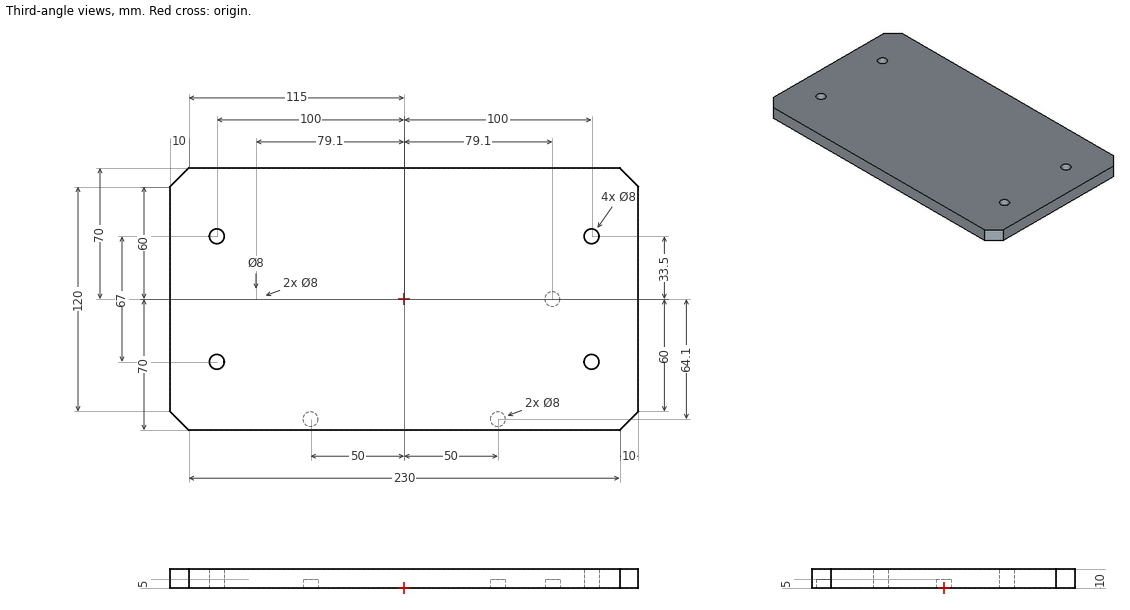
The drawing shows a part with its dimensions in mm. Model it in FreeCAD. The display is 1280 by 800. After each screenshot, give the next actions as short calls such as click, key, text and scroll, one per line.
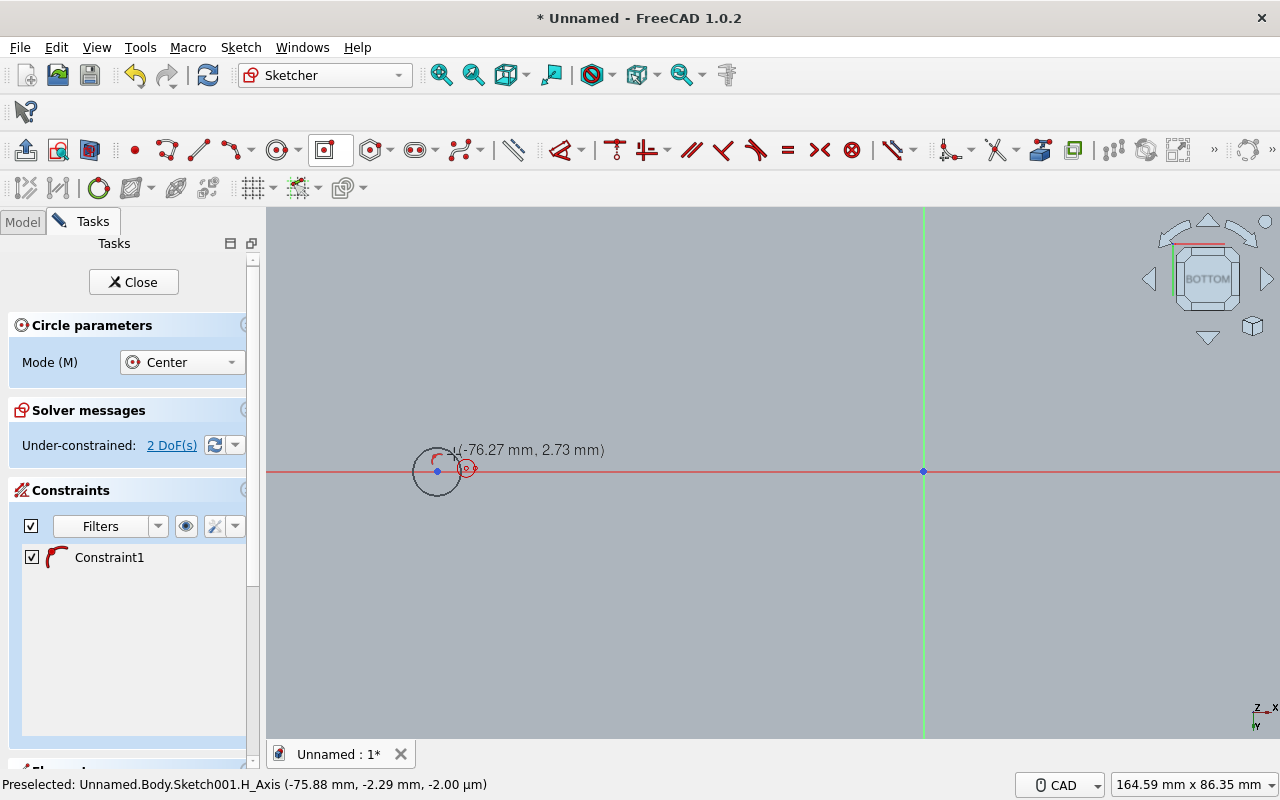
scroll(438, 474, down, 3)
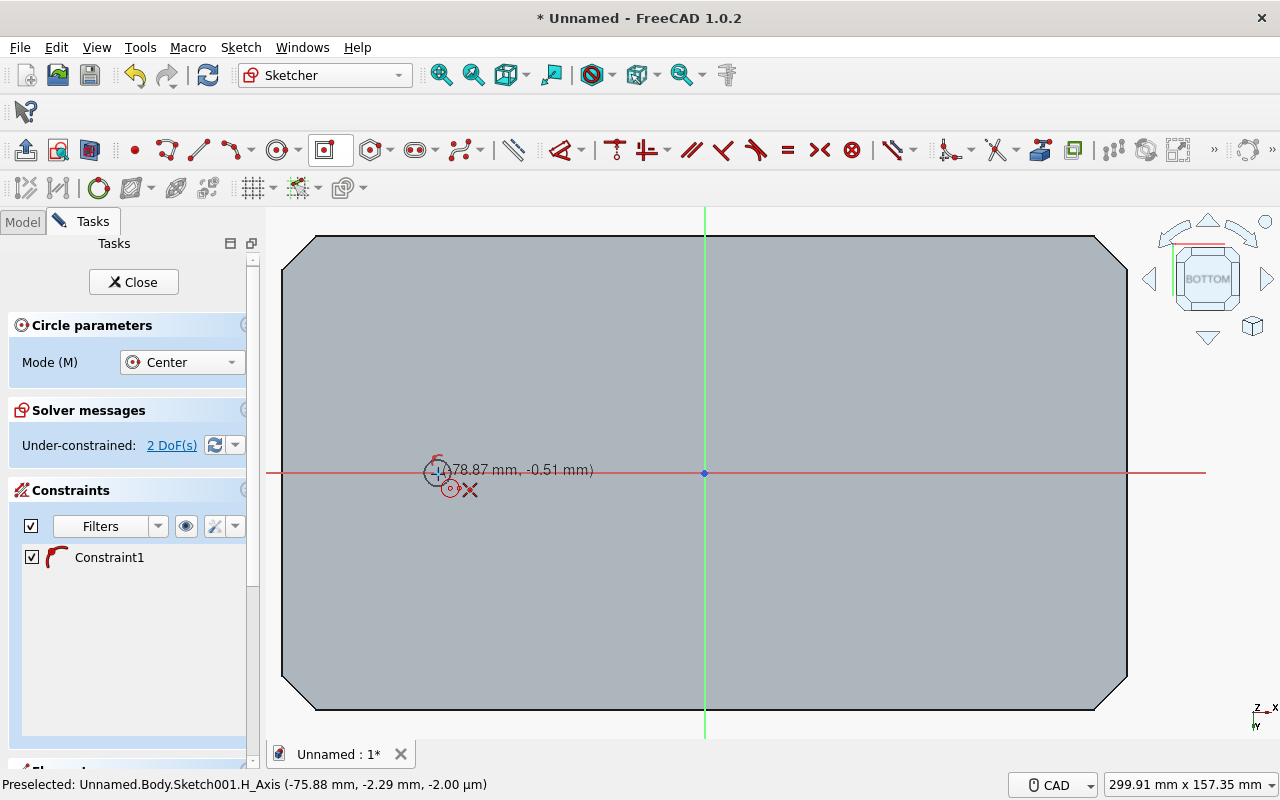
scroll(972, 473, up, 3)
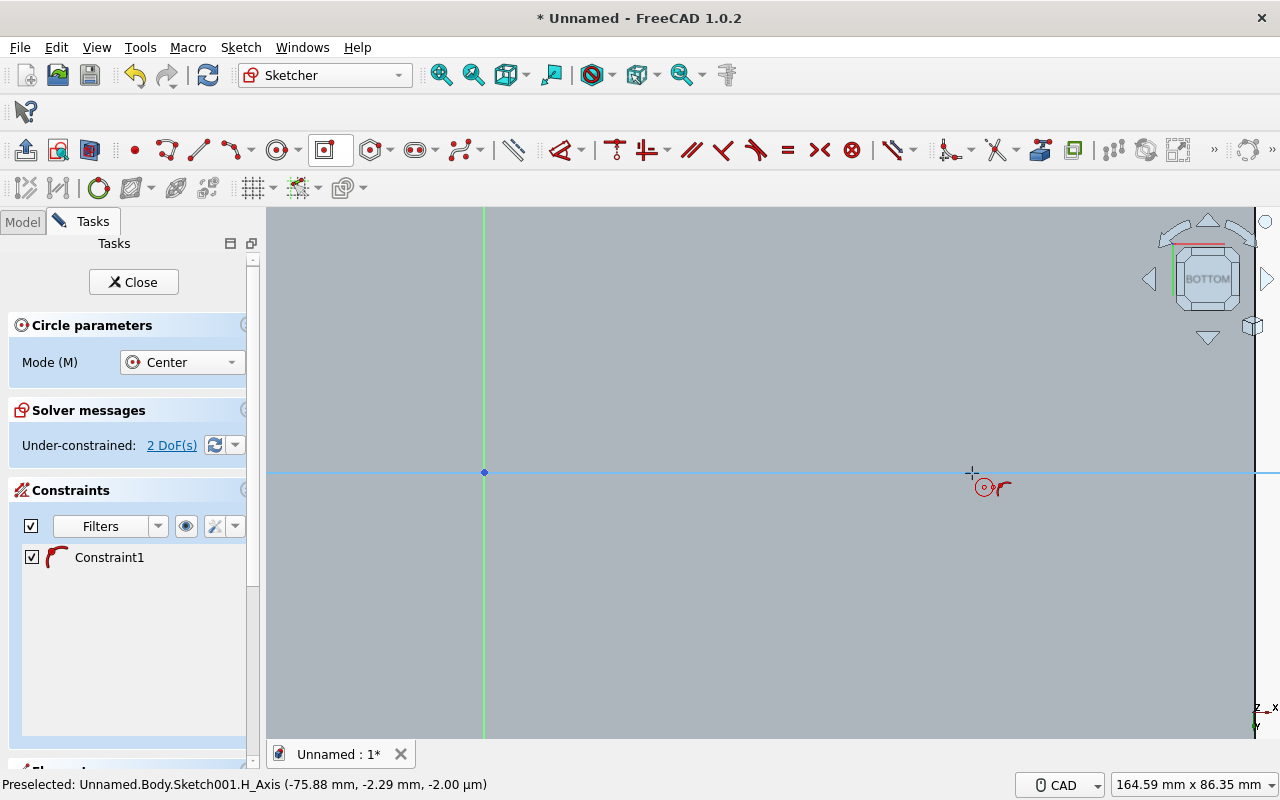
click(972, 473)
click(989, 455)
key(Escape)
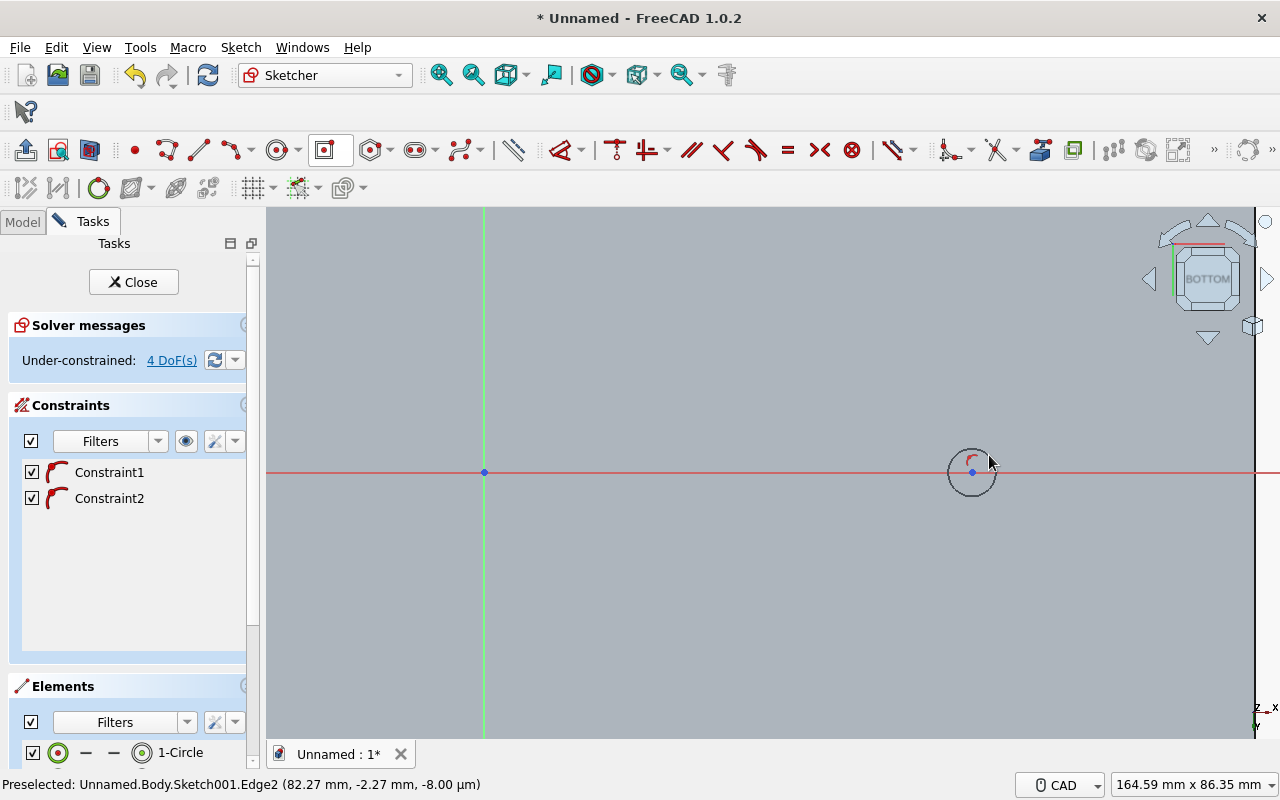
scroll(972, 473, down, 3)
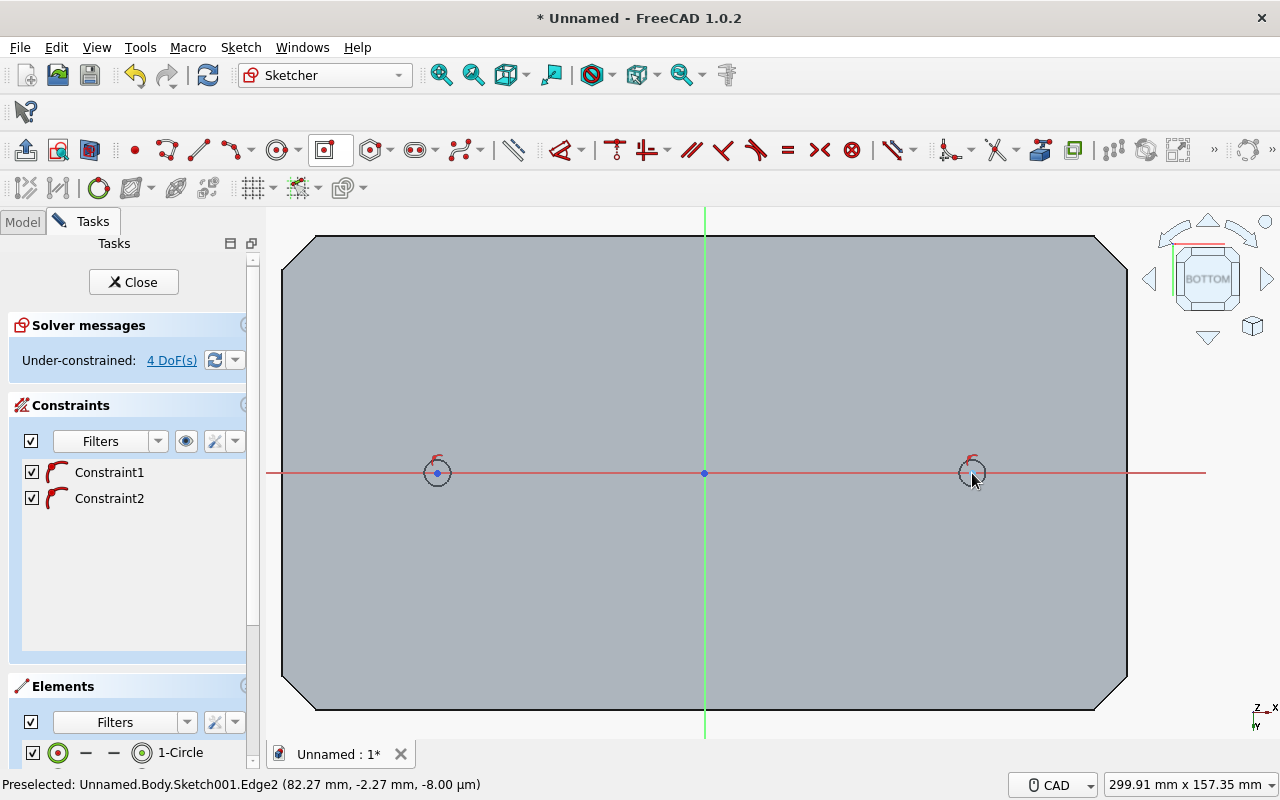
scroll(447, 464, up, 2)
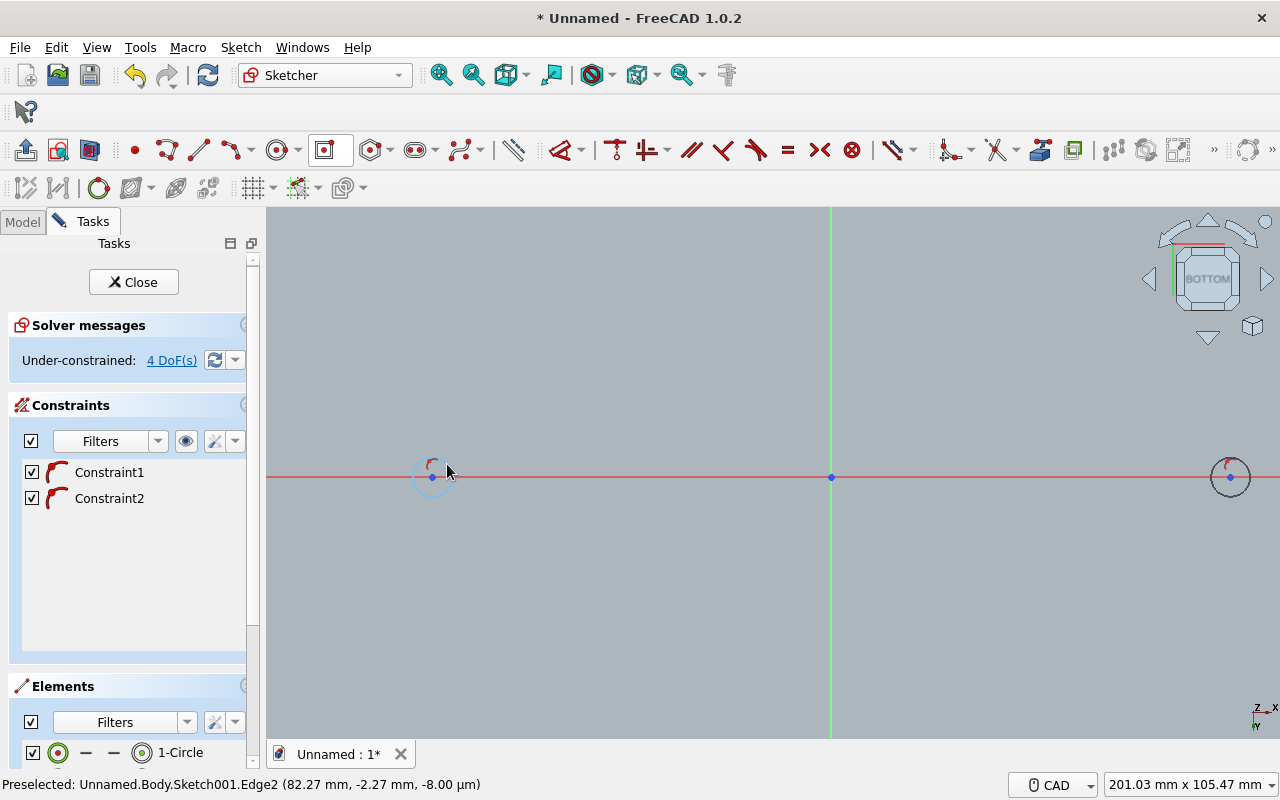
click(447, 463)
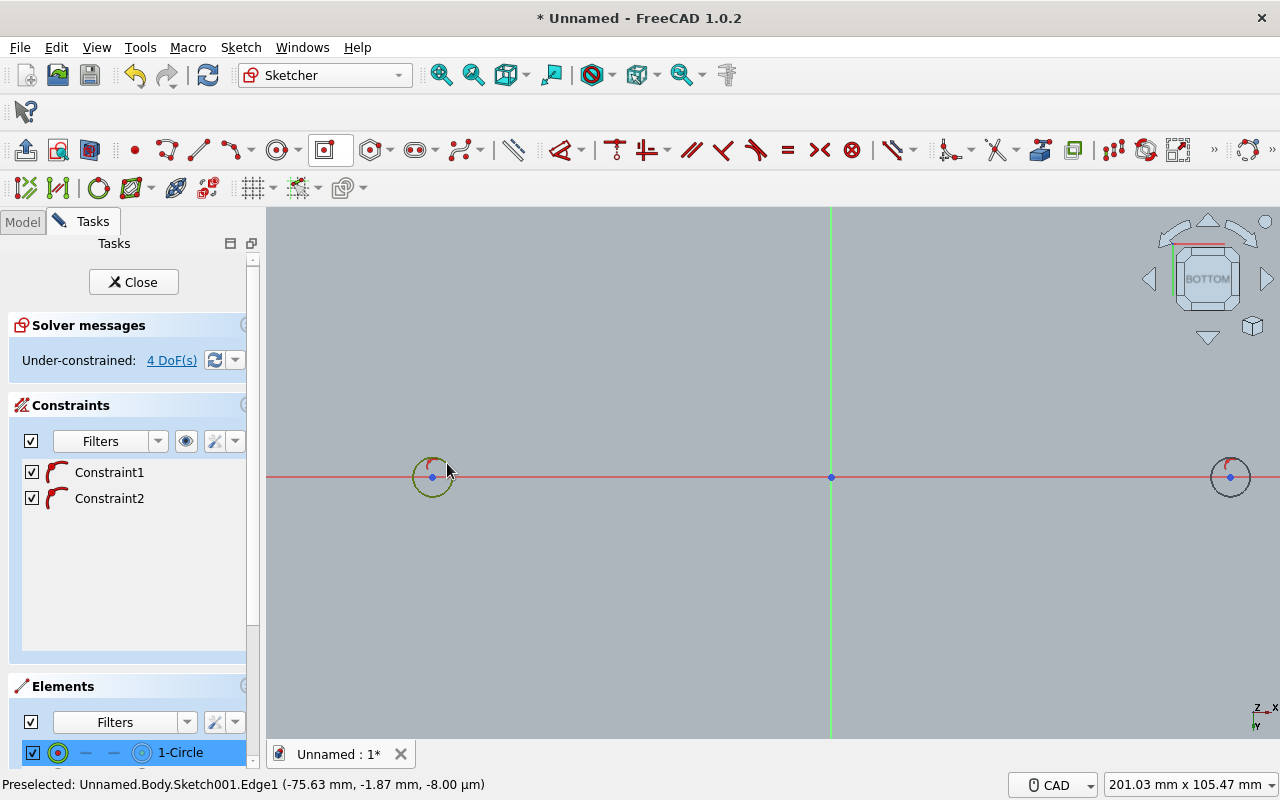
scroll(446, 464, down, 2)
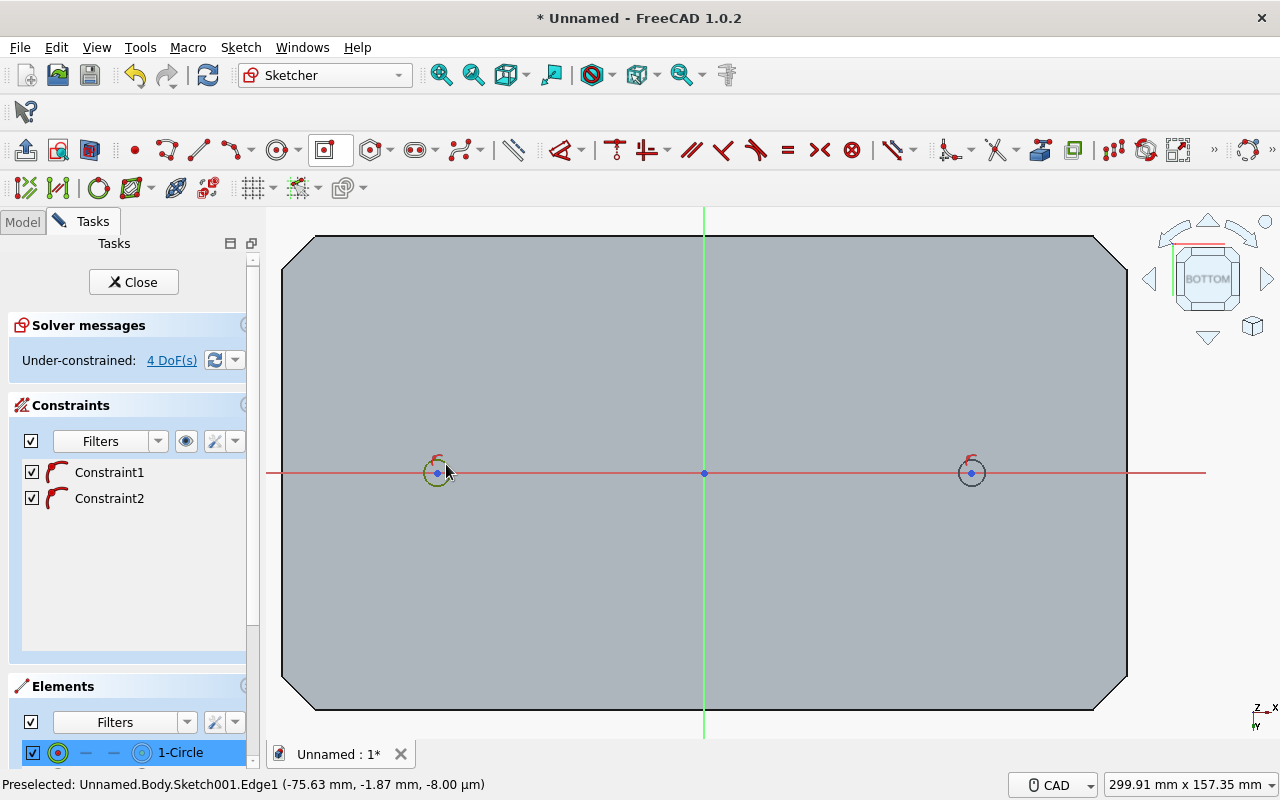
scroll(981, 464, up, 2)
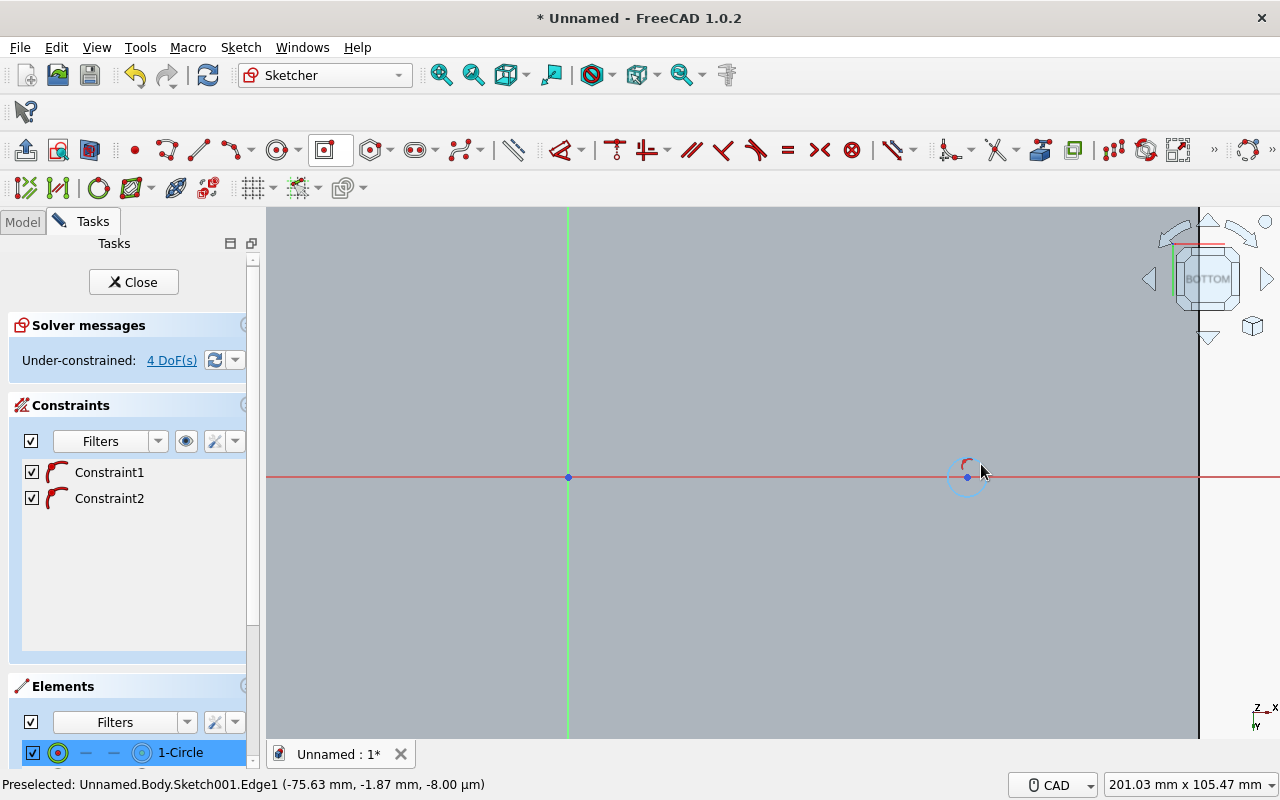
click(981, 463)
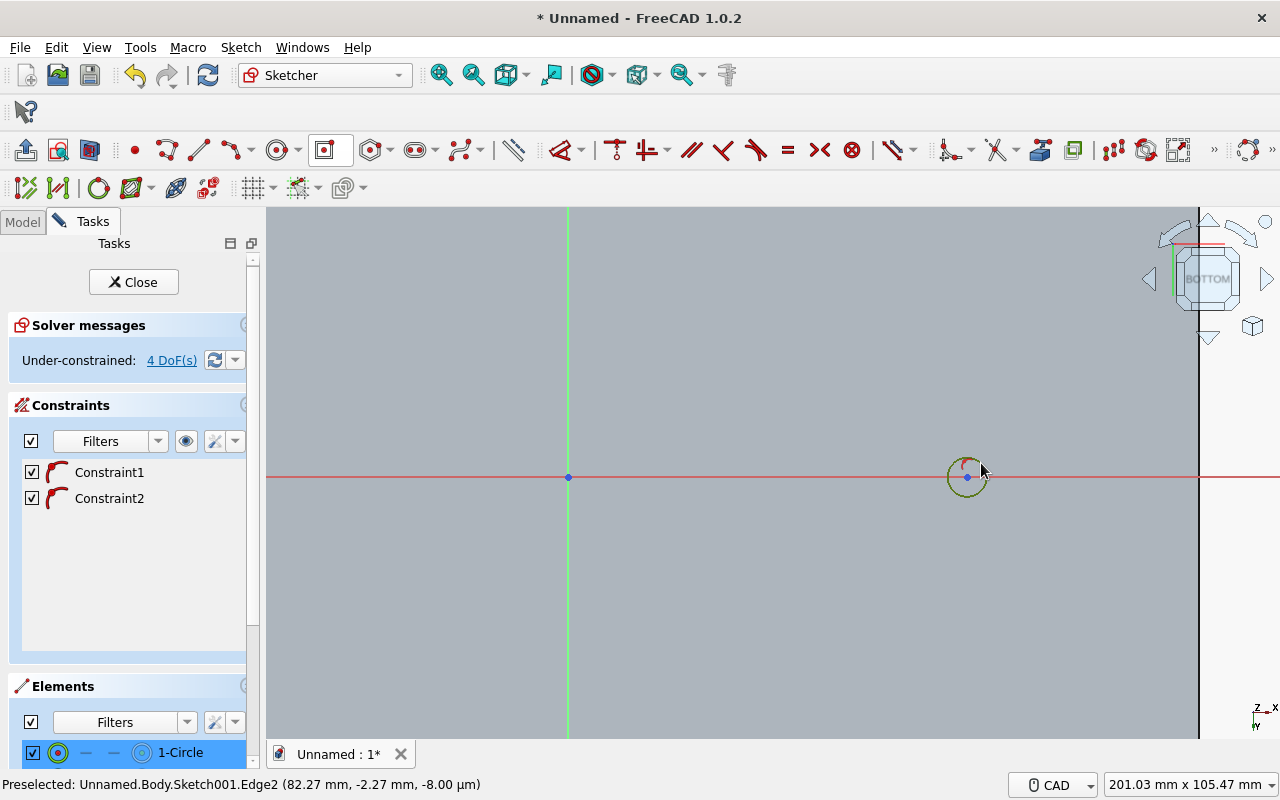
click(788, 150)